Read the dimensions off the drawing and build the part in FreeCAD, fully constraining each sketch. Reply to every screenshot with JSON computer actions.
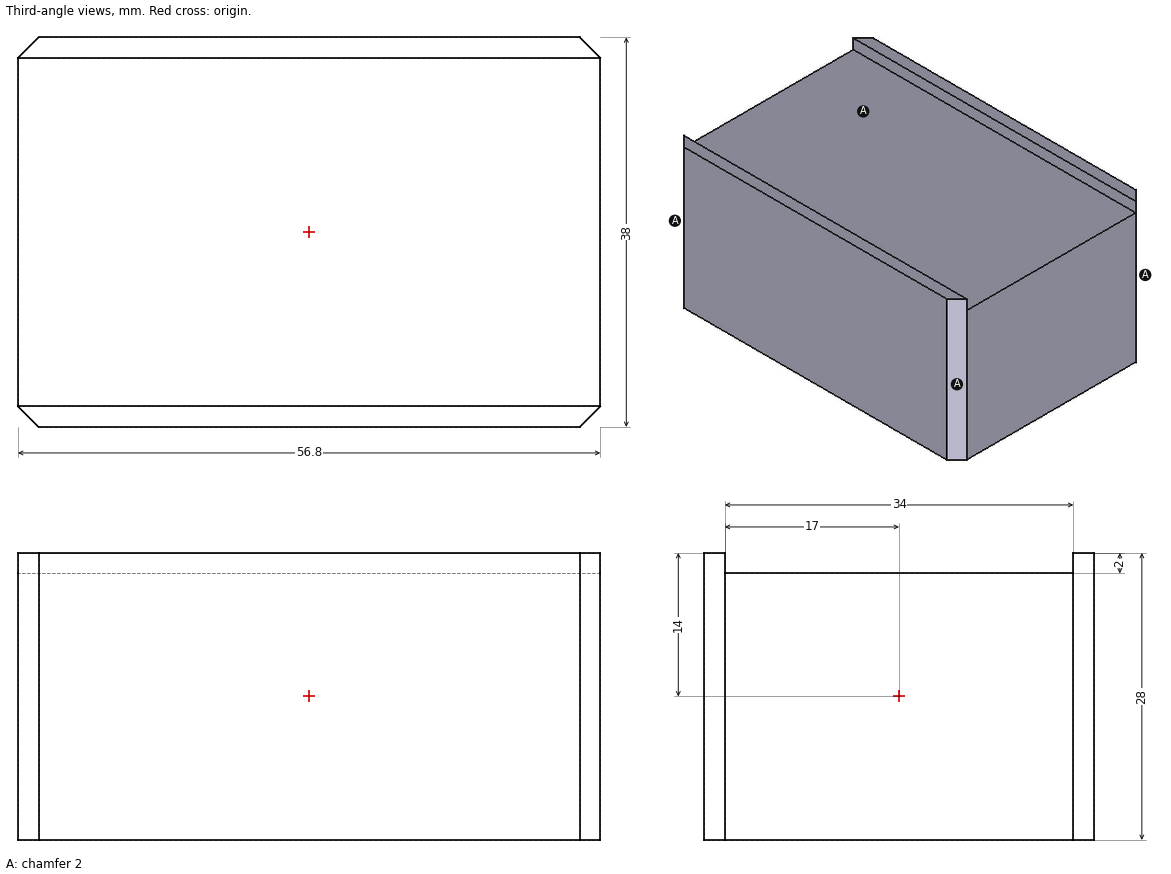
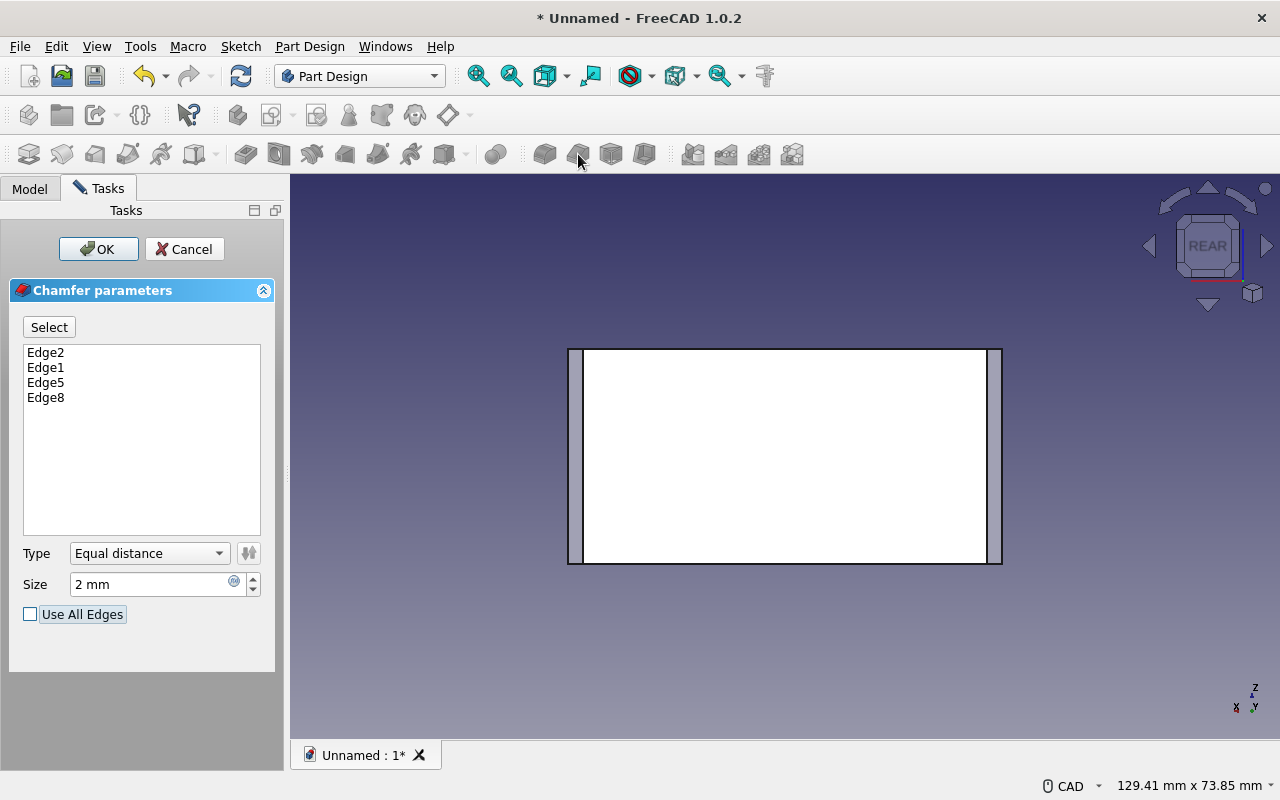
{"action": "left_click", "coordinate": [99, 249]}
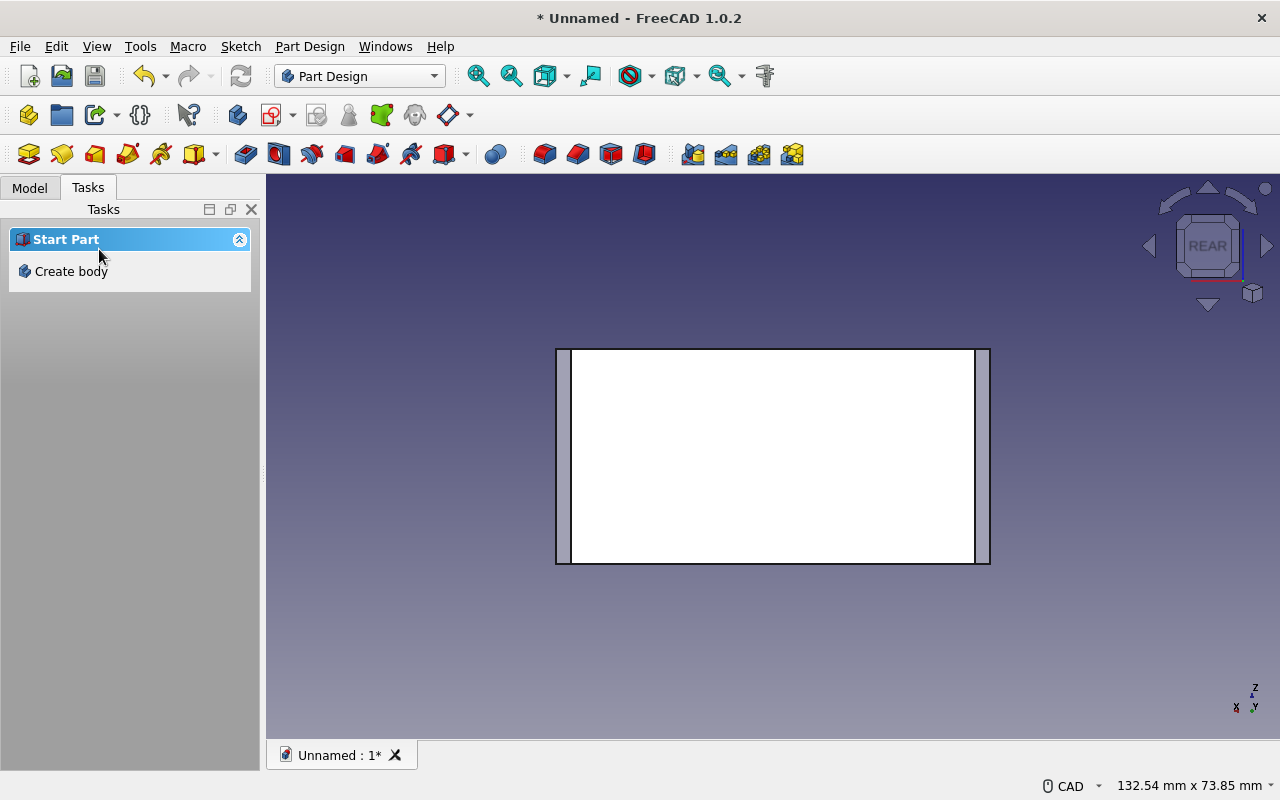
{"action": "left_click", "coordinate": [479, 76]}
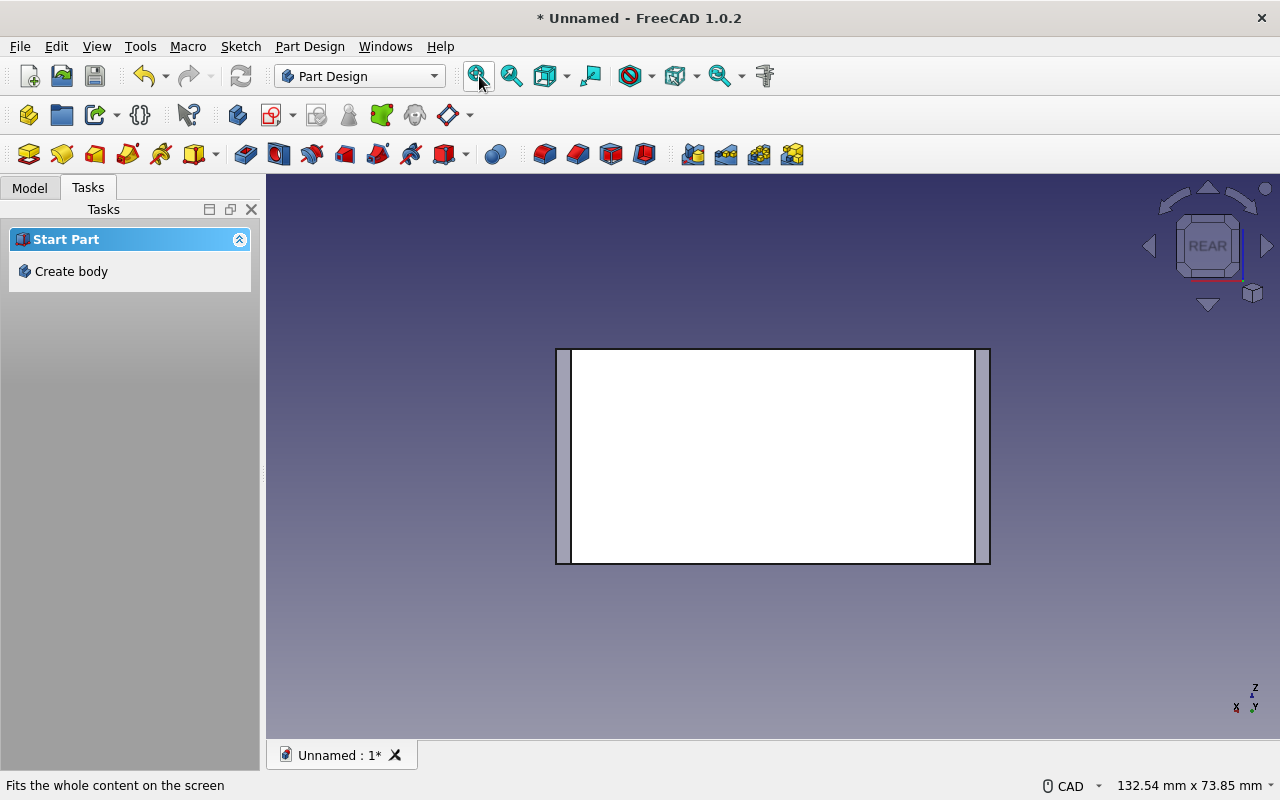
{"action": "key", "text": "0"}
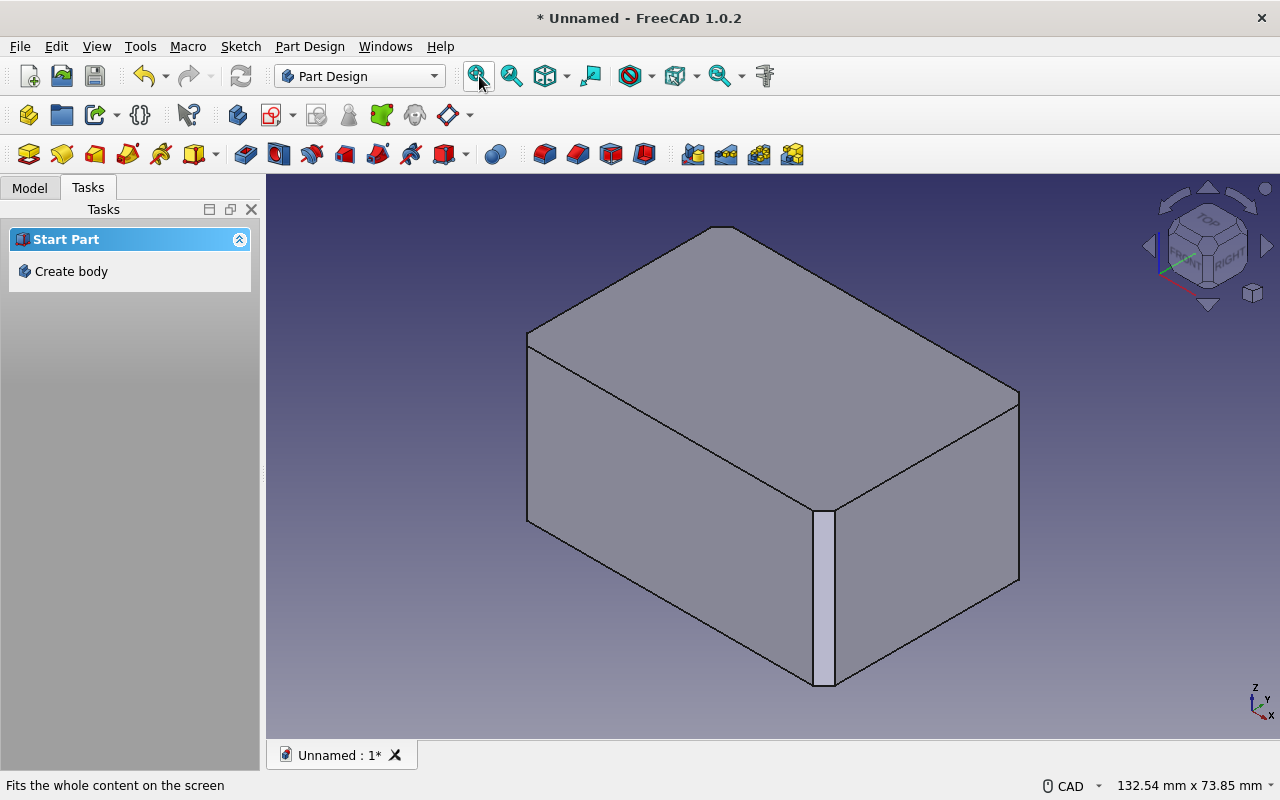
{"action": "left_click", "coordinate": [927, 544]}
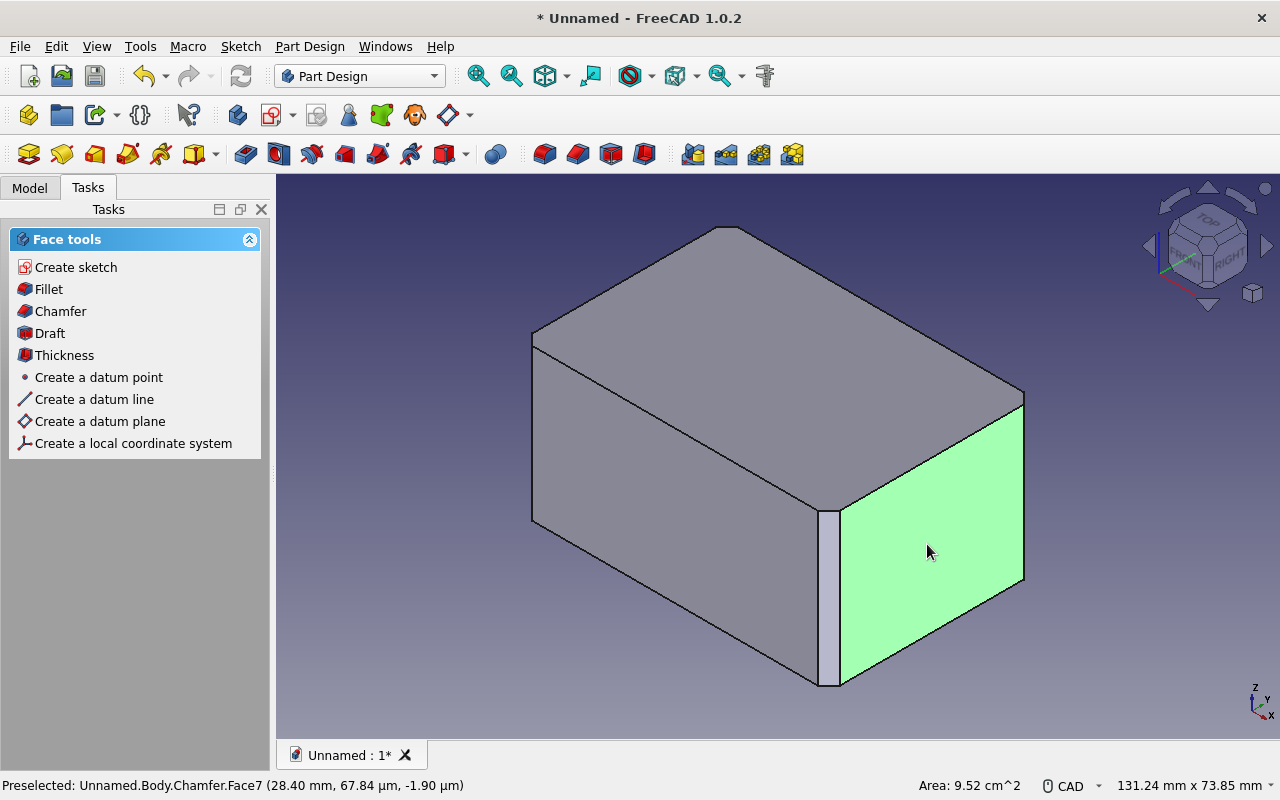
{"action": "left_click", "coordinate": [270, 116]}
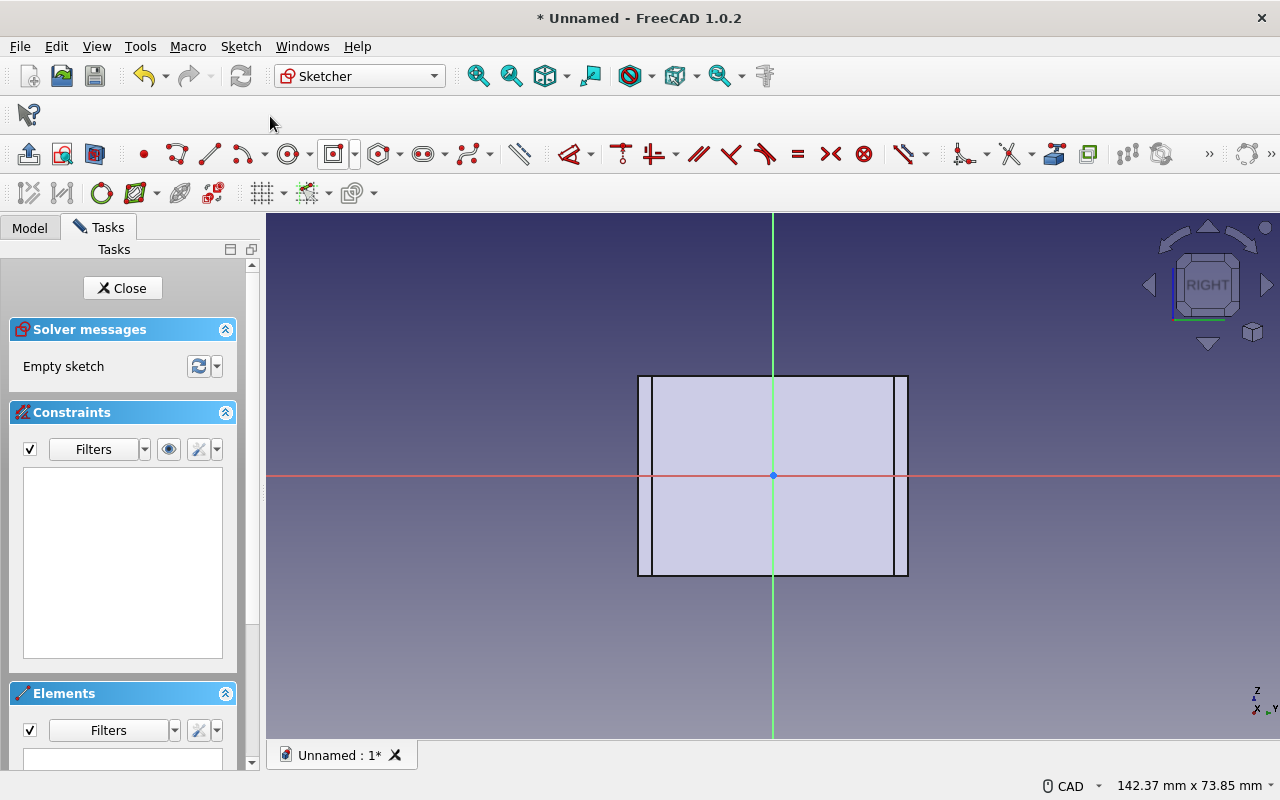
{"action": "scroll", "coordinate": [829, 385], "scroll_direction": "up", "scroll_amount": 4}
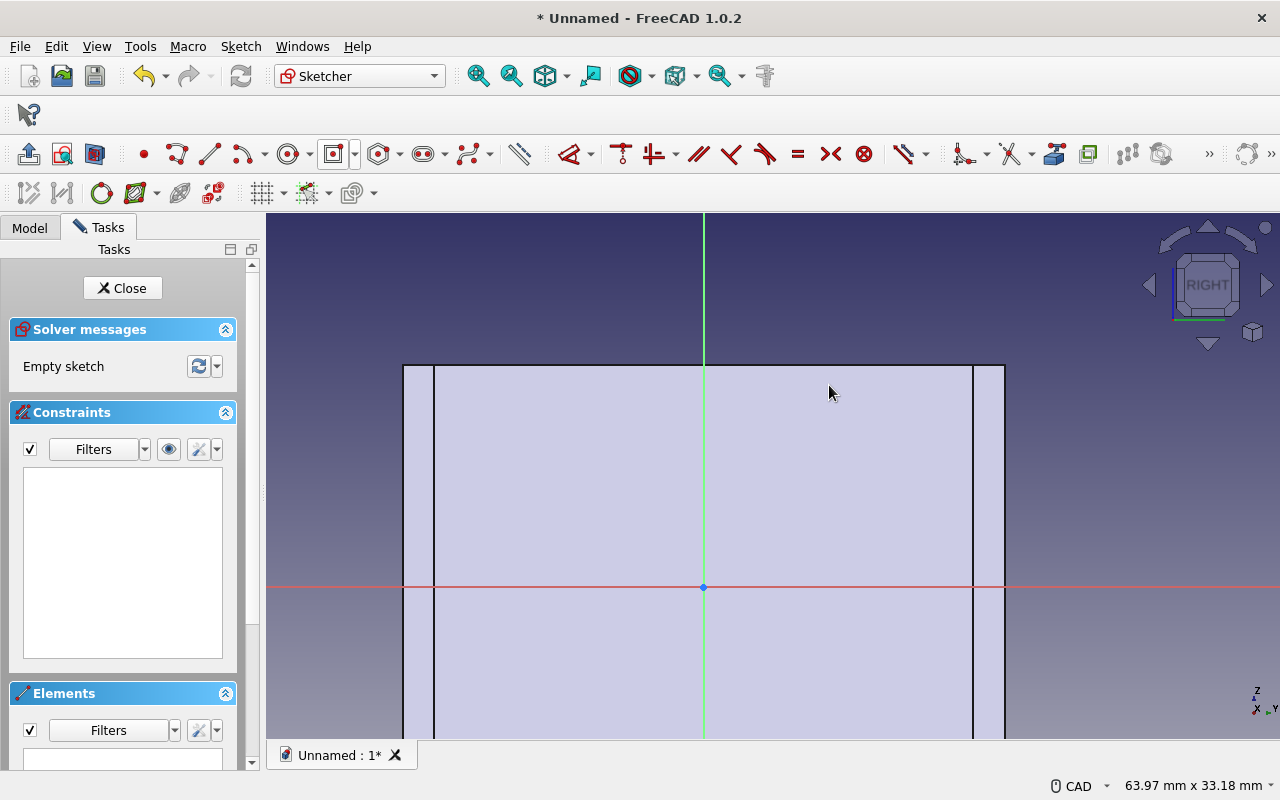
{"action": "key", "text": "g r"}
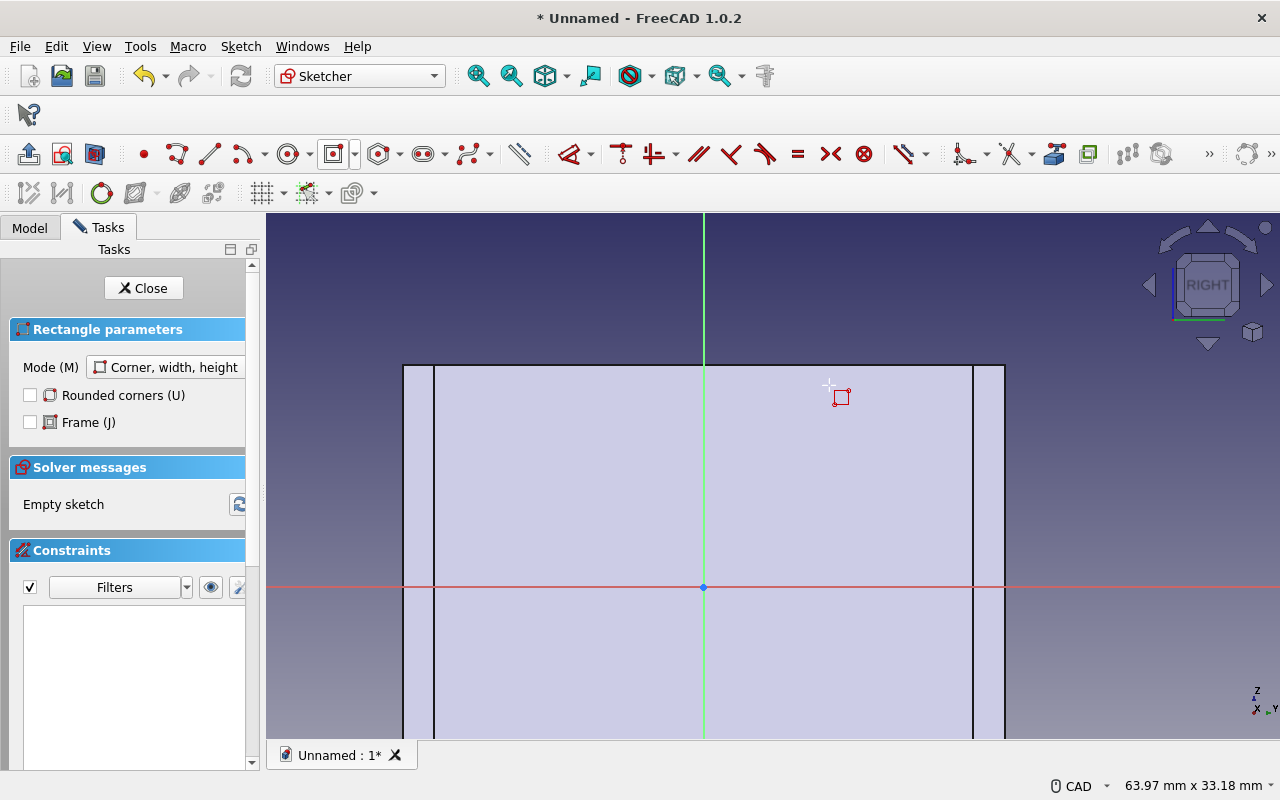
{"action": "left_click", "coordinate": [434, 365]}
{"action": "mouse_move", "coordinate": [973, 397]}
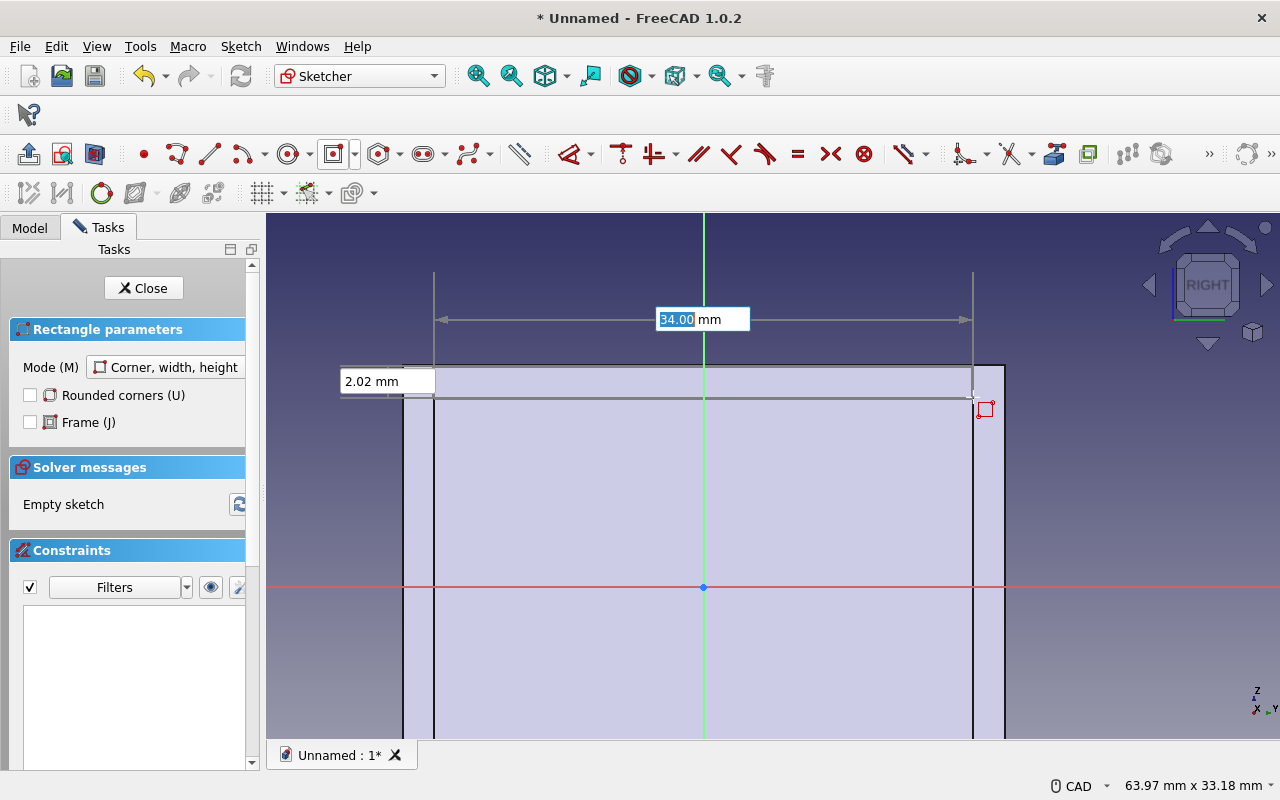
{"action": "type", "text": "34"}
{"action": "key", "text": "Tab"}
{"action": "type", "text": "2"}
{"action": "key", "text": "Return"}
{"action": "key", "text": "Escape"}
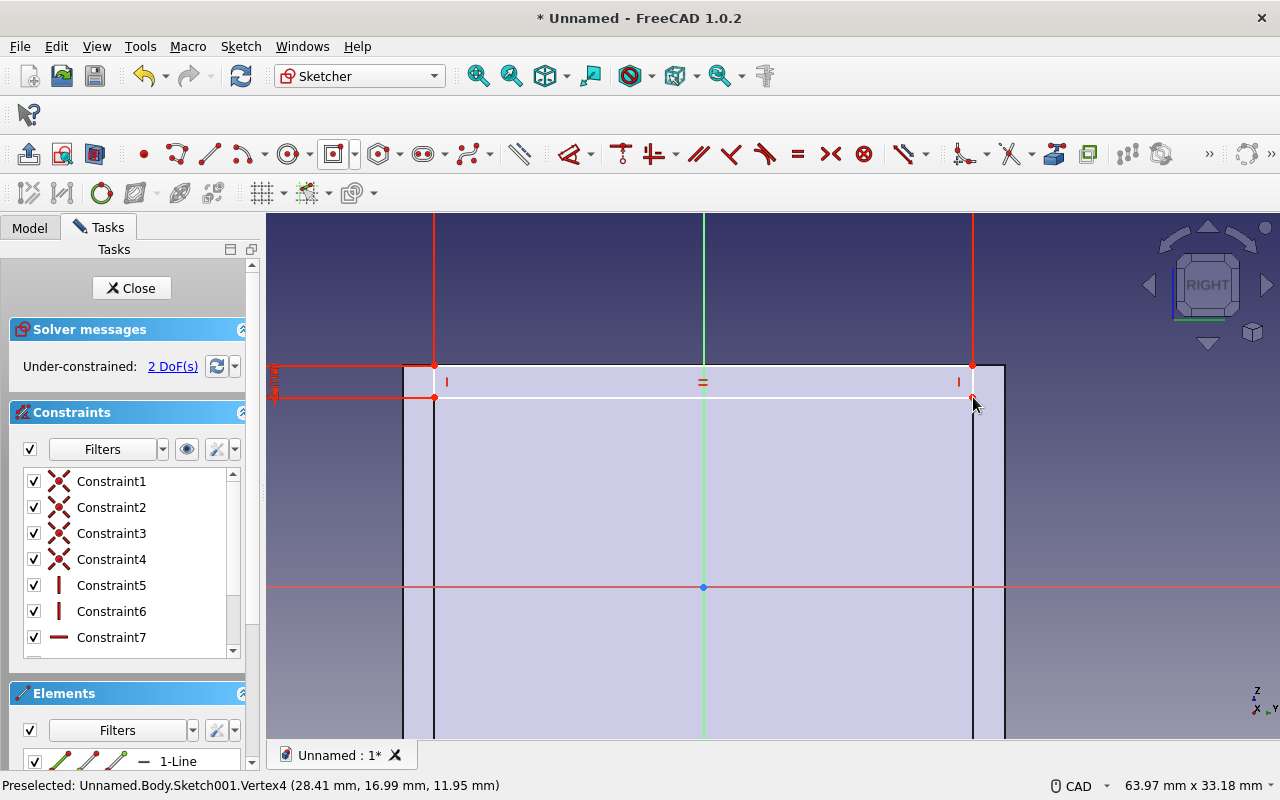
{"action": "left_click", "coordinate": [568, 154]}